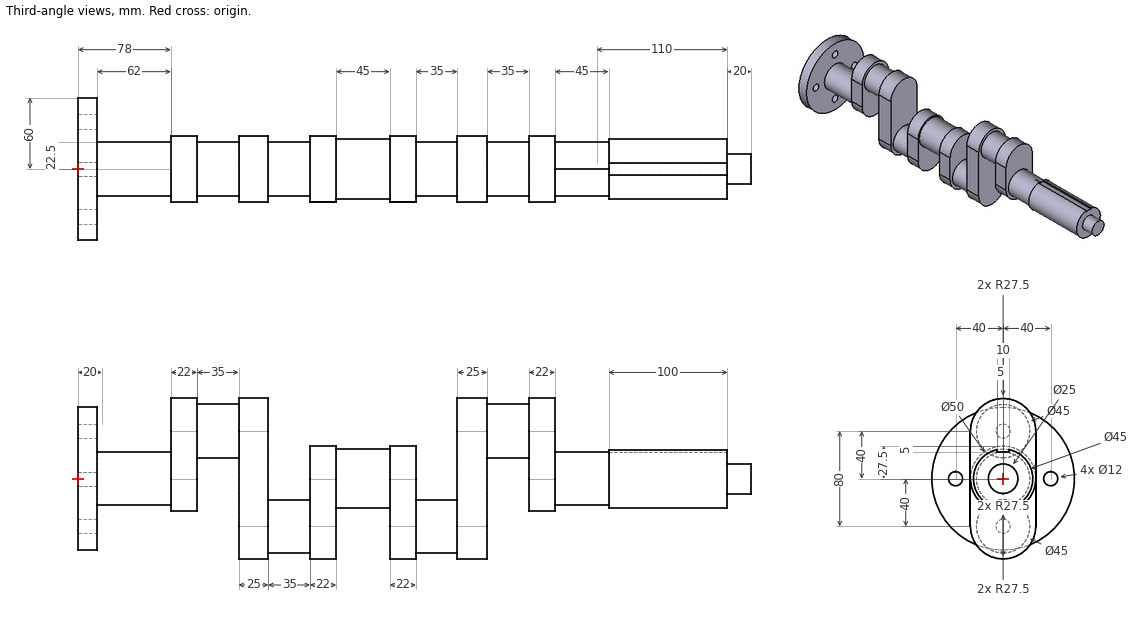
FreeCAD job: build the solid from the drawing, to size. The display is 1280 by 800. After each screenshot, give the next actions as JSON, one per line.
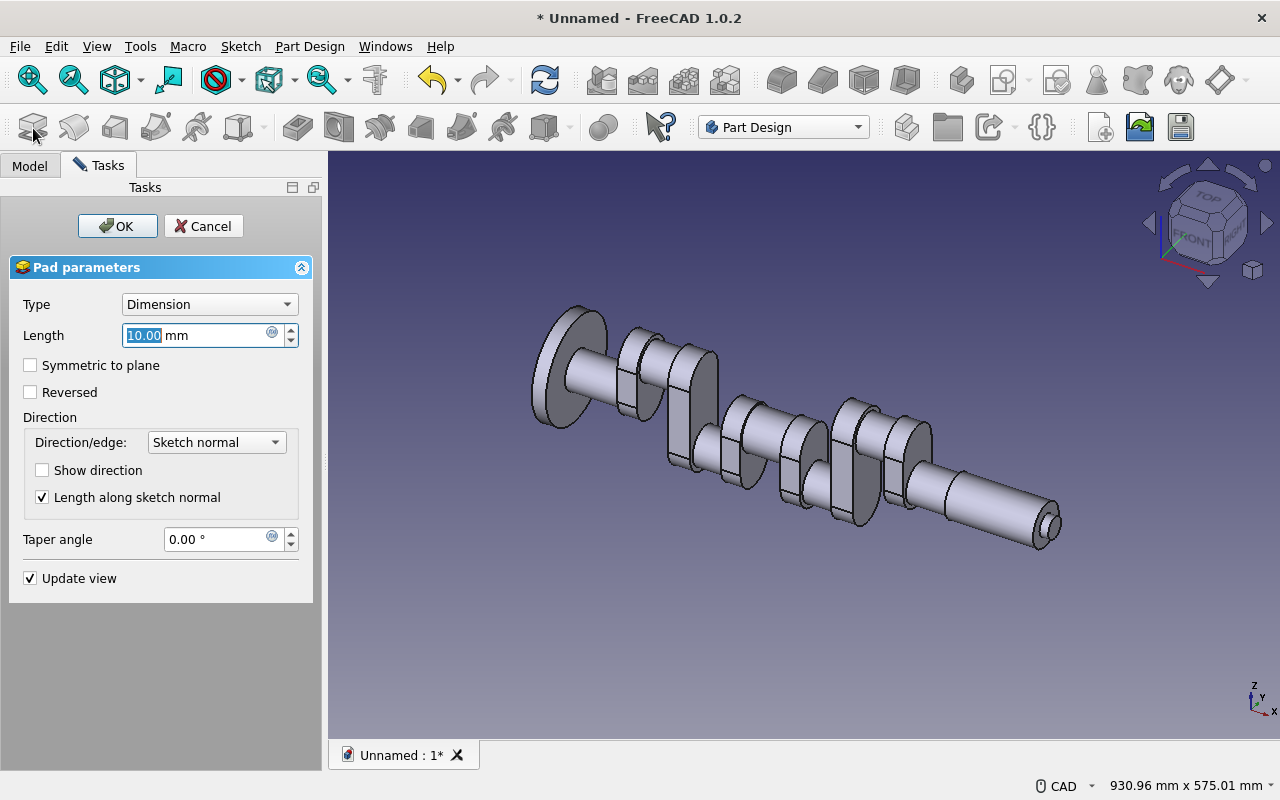
{"action": "type", "text": "20"}
{"action": "key", "text": "Tab"}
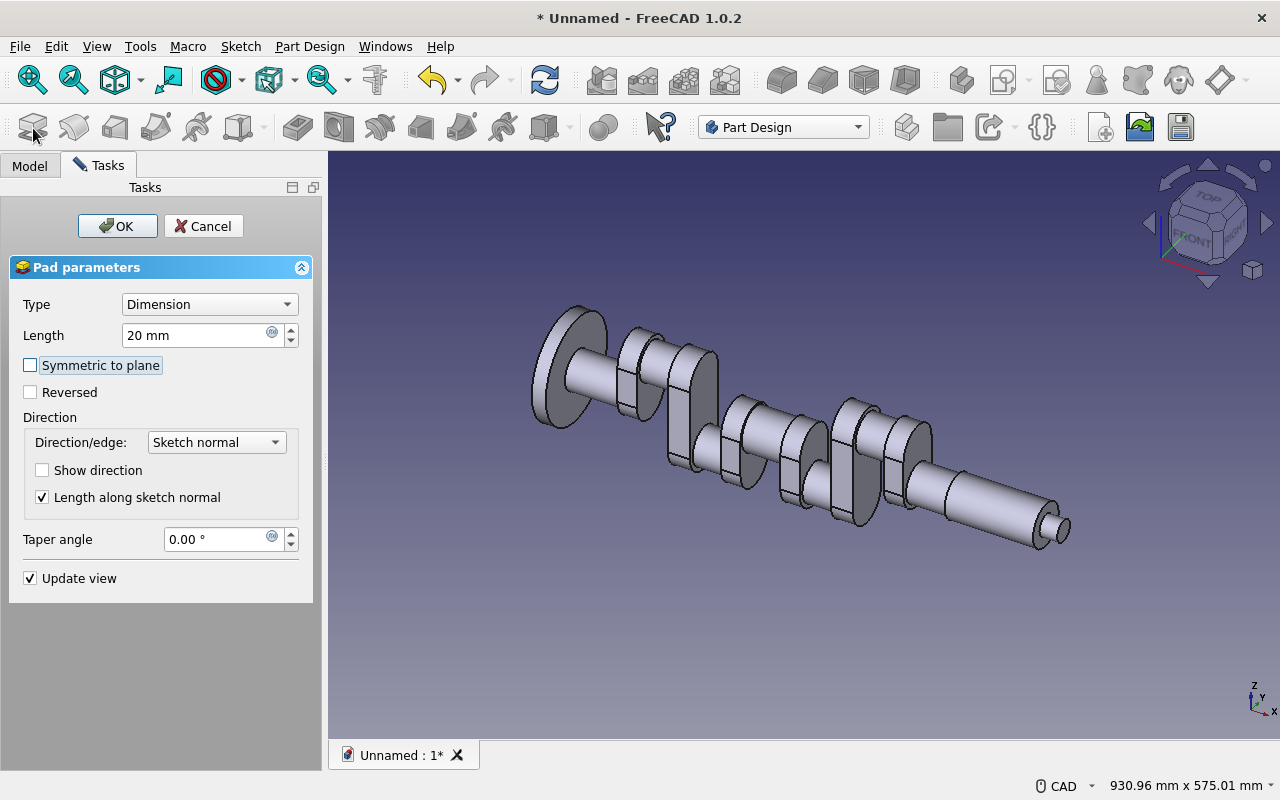
{"action": "left_click", "coordinate": [118, 226]}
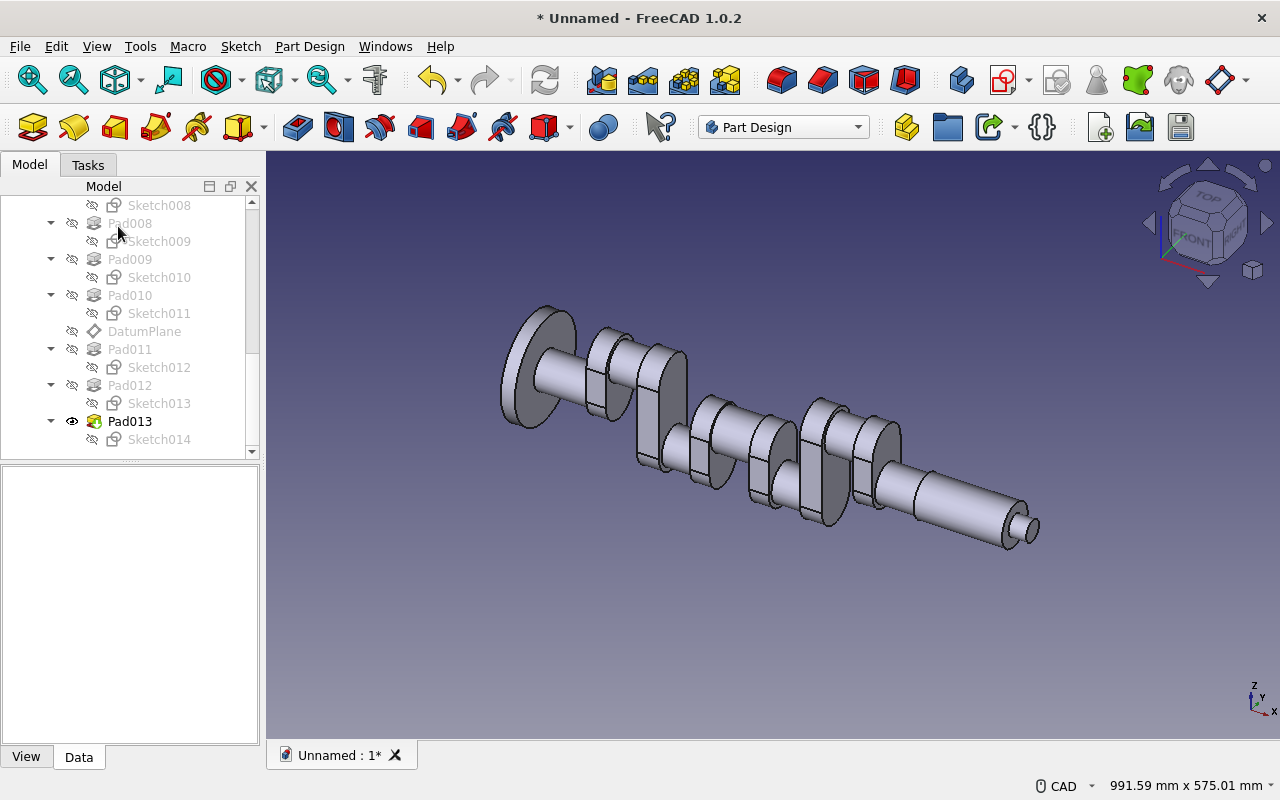
{"action": "key", "text": "6"}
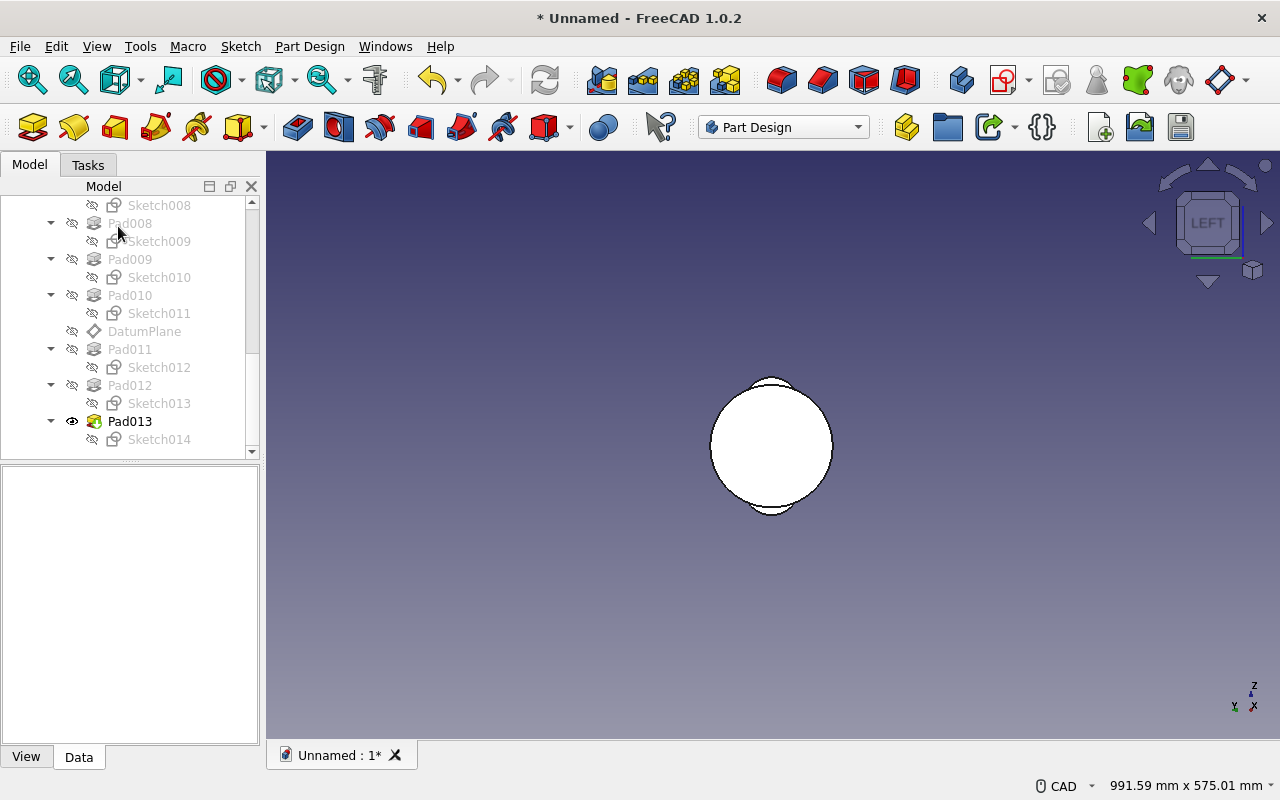
{"action": "left_click", "coordinate": [33, 80]}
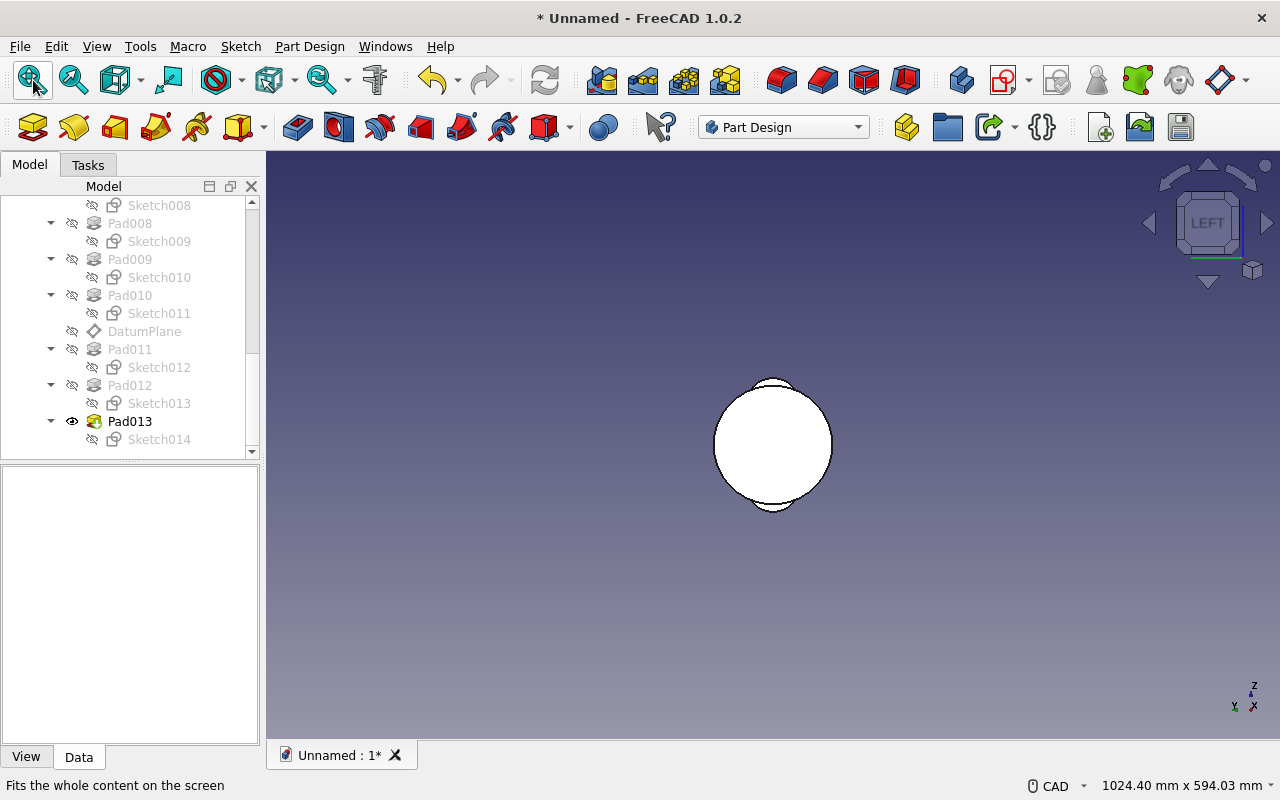
{"action": "left_click", "coordinate": [773, 444]}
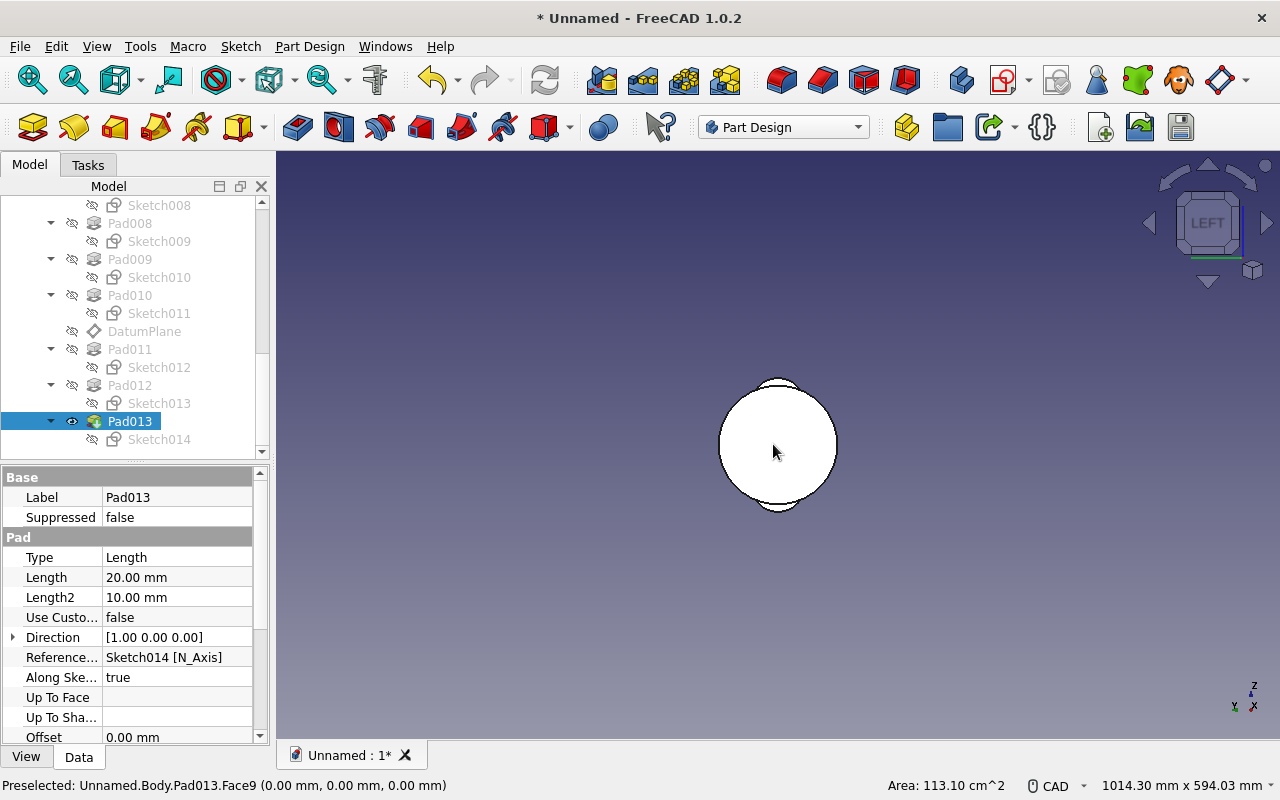
{"action": "left_click", "coordinate": [1002, 80]}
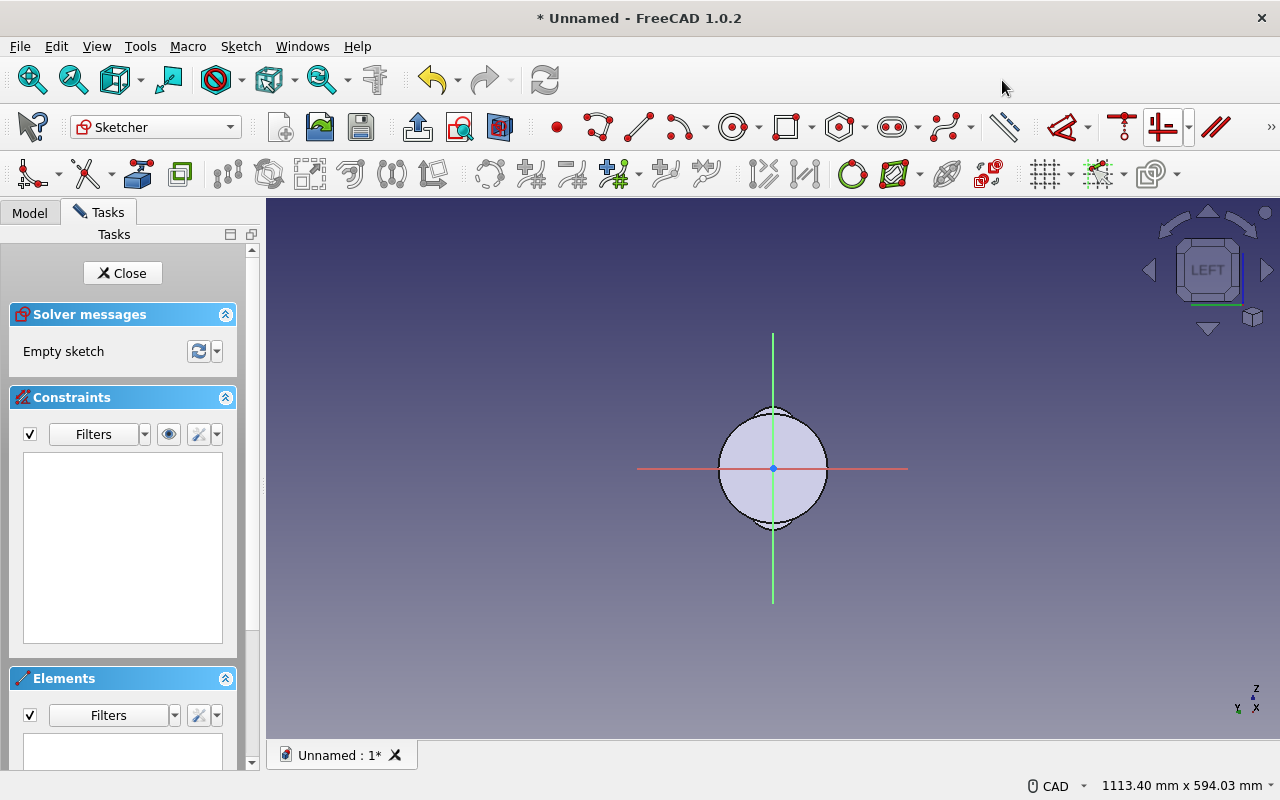
{"action": "scroll", "coordinate": [795, 468], "scroll_direction": "up", "scroll_amount": 7}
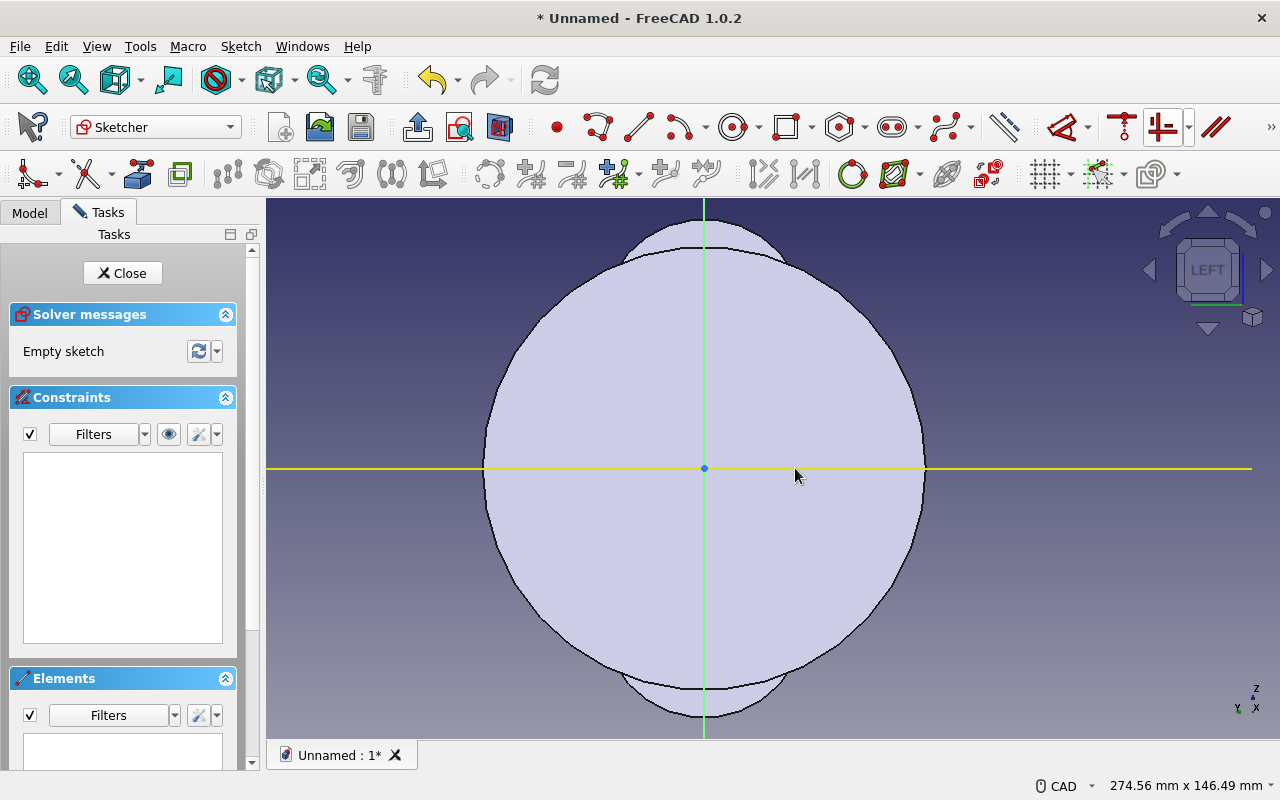
{"action": "left_click", "coordinate": [732, 128]}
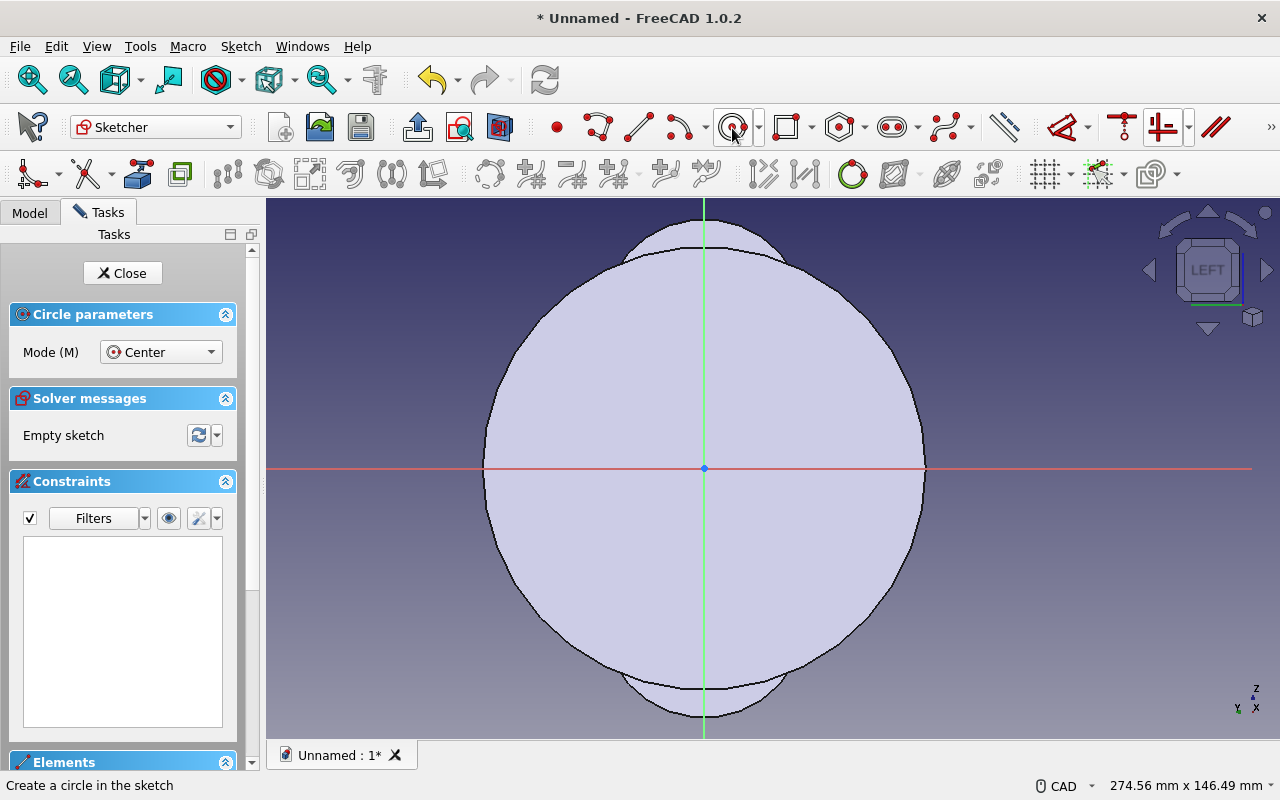
{"action": "left_click", "coordinate": [556, 468]}
{"action": "left_click", "coordinate": [572, 453]}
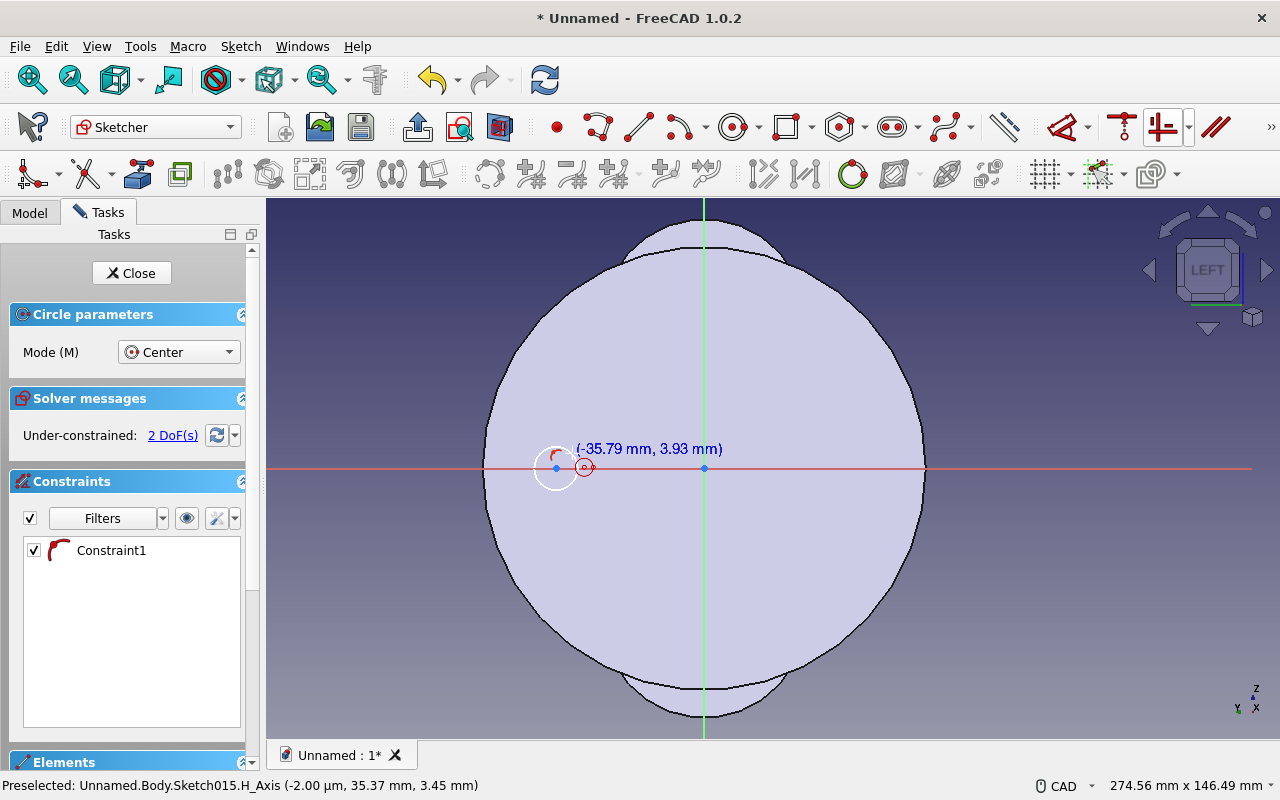
{"action": "left_click", "coordinate": [704, 321]}
{"action": "left_click", "coordinate": [720, 305]}